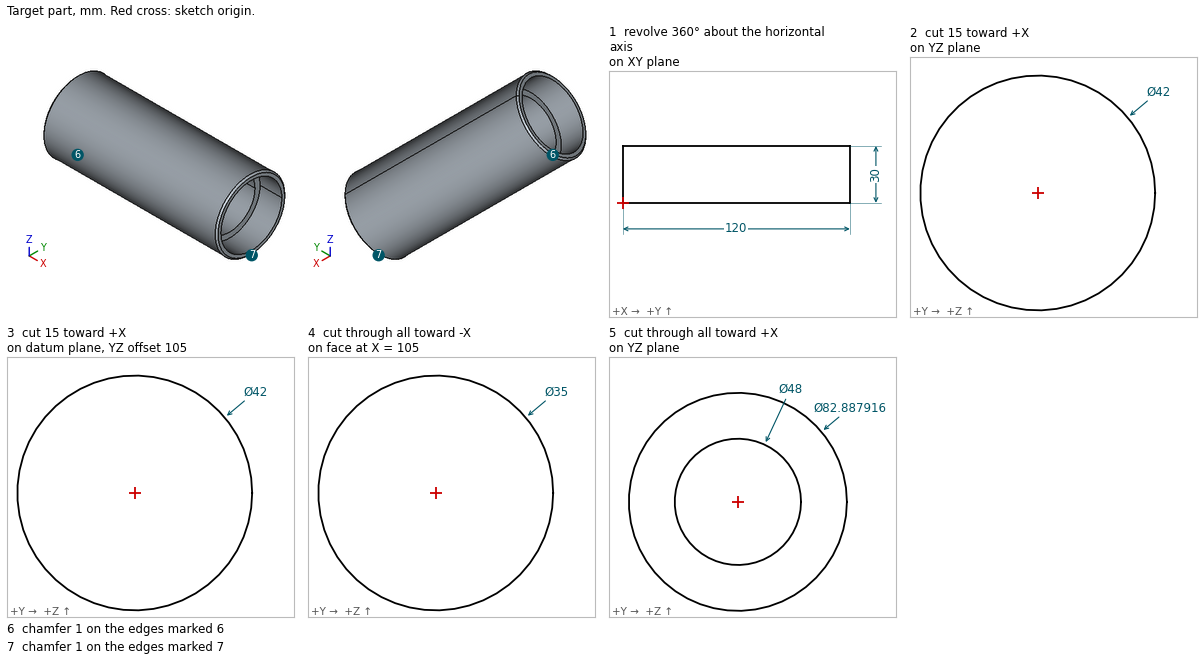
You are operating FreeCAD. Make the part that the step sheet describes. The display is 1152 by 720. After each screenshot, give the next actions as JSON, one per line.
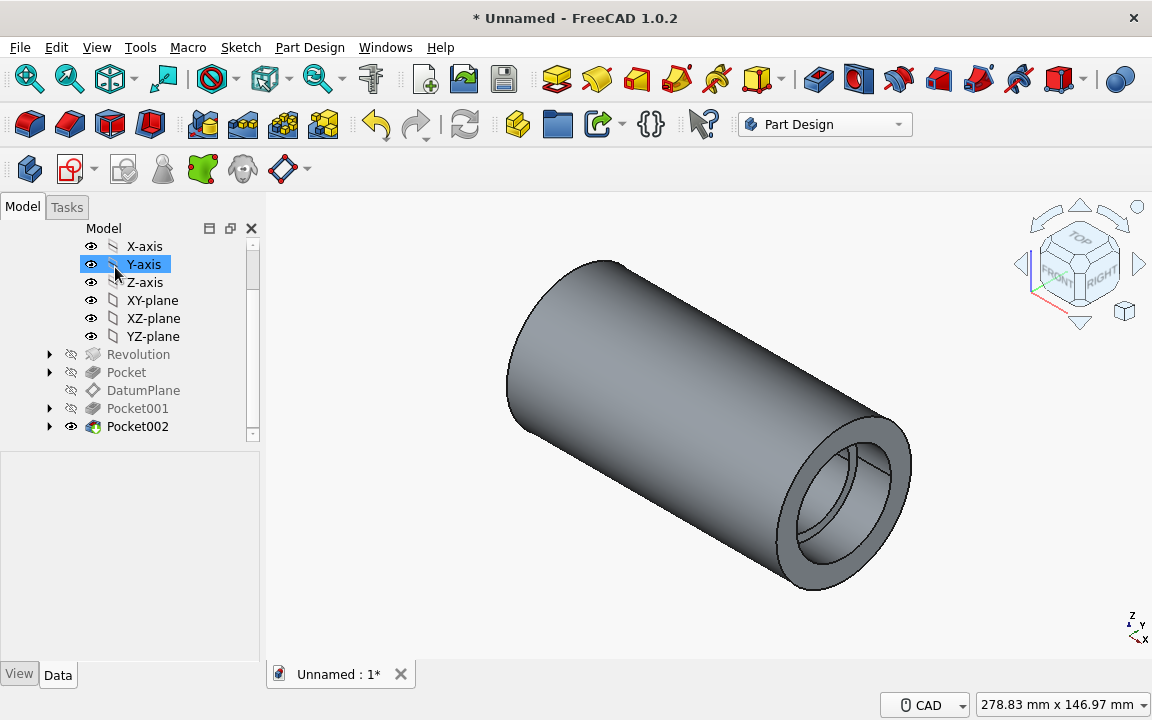
{"action": "left_click", "coordinate": [70, 170]}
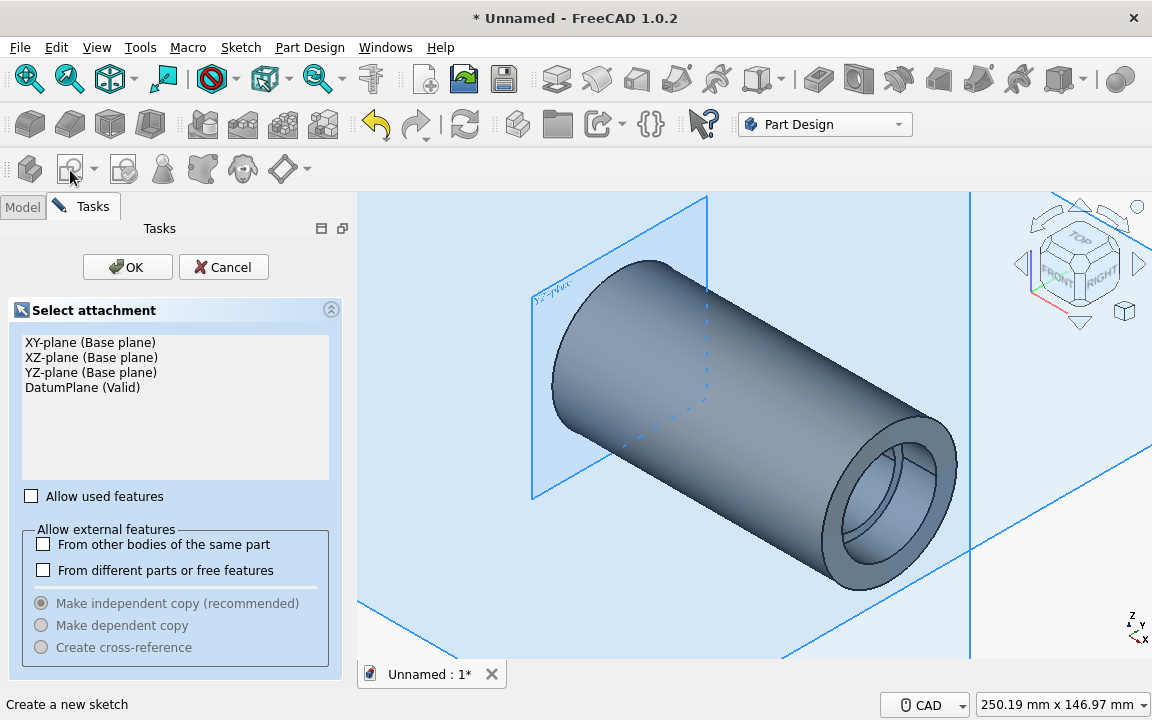
{"action": "left_click", "coordinate": [82, 372]}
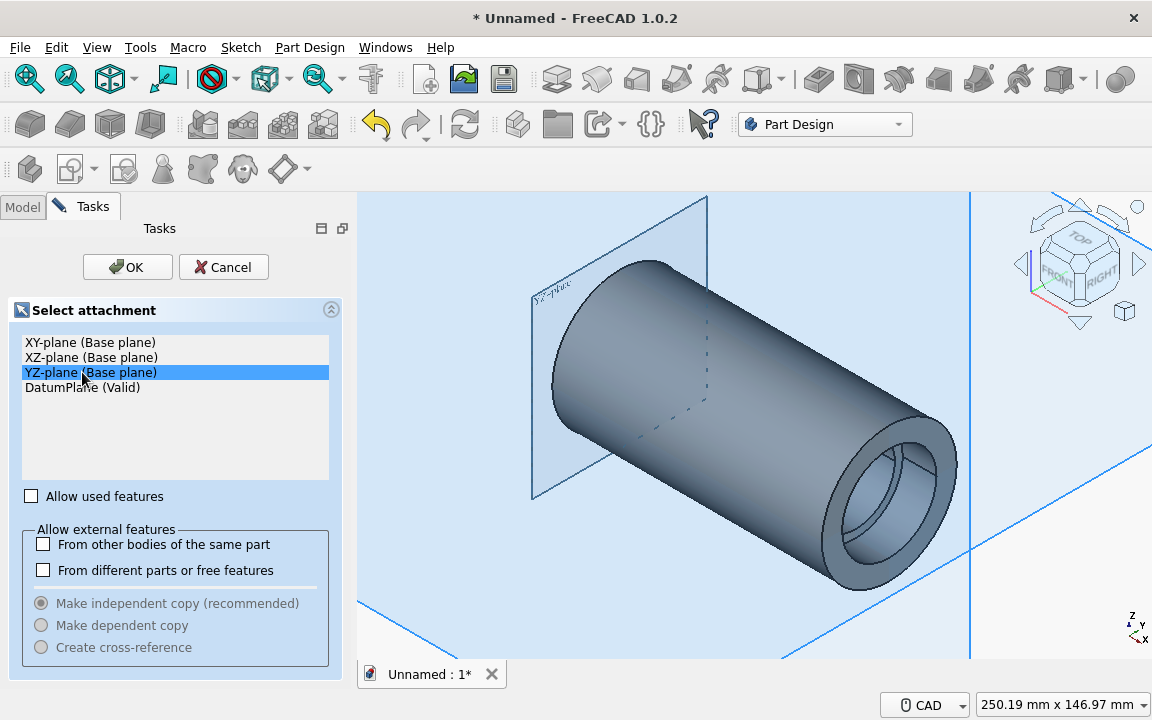
{"action": "left_click", "coordinate": [128, 267]}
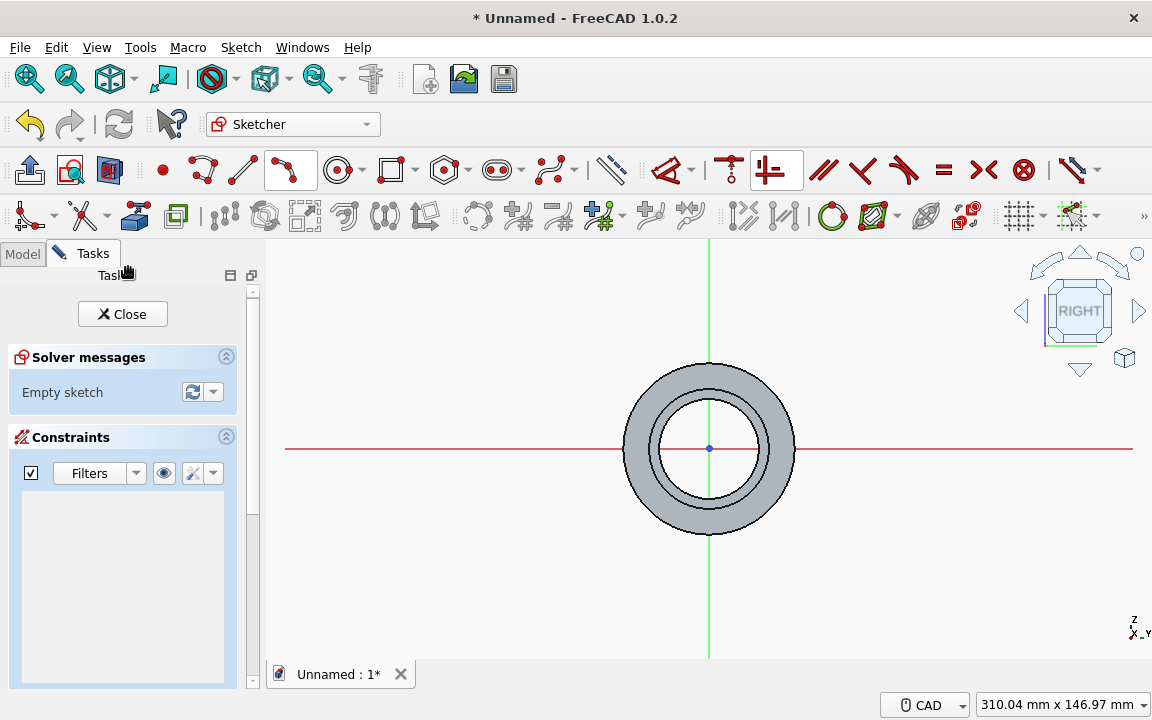
{"action": "key", "text": "q s"}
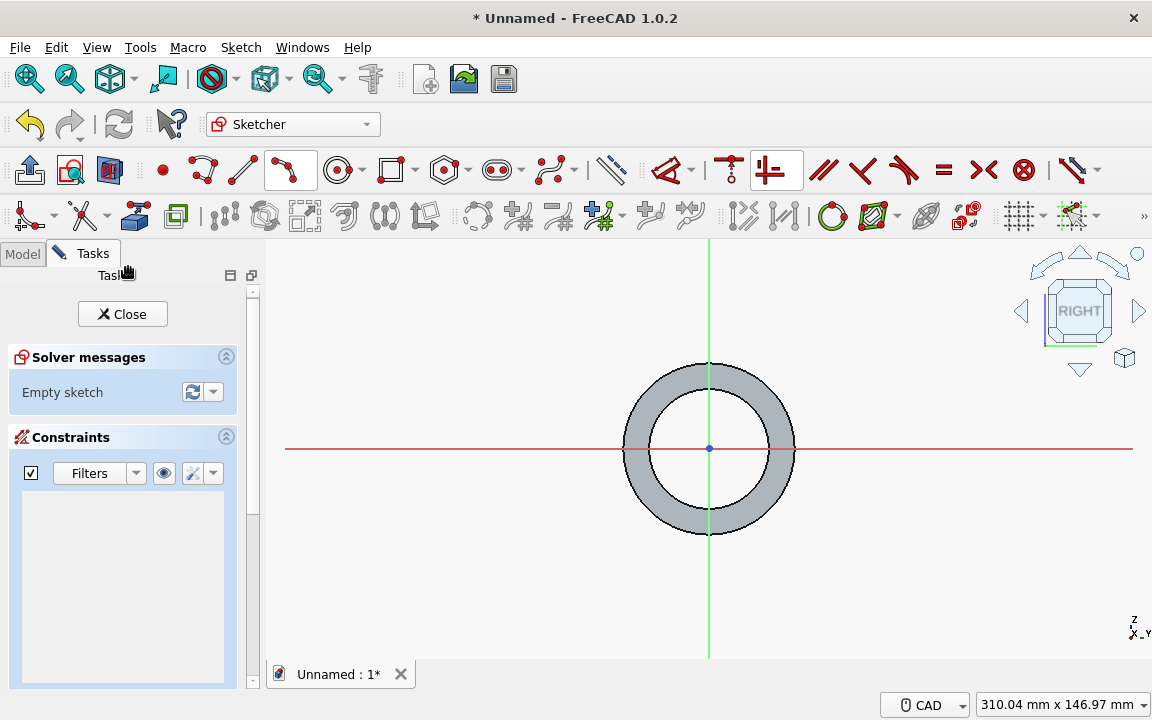
{"action": "key", "text": "g c"}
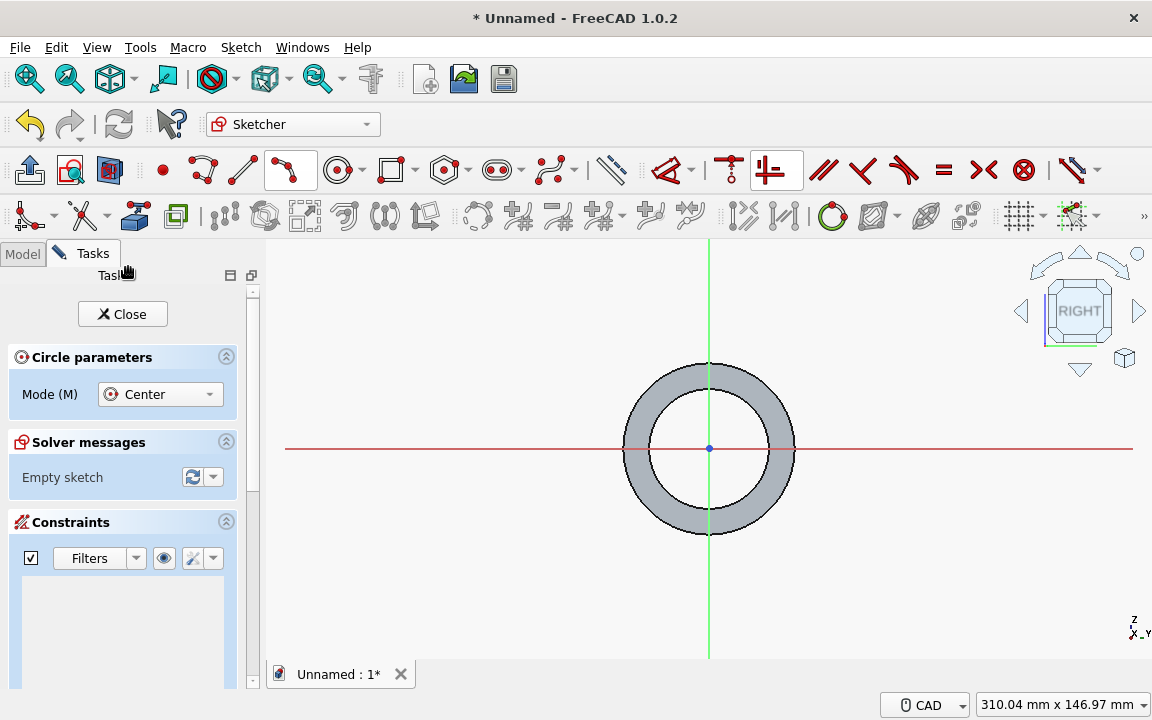
{"action": "left_click", "coordinate": [709, 449]}
{"action": "left_click", "coordinate": [793, 365]}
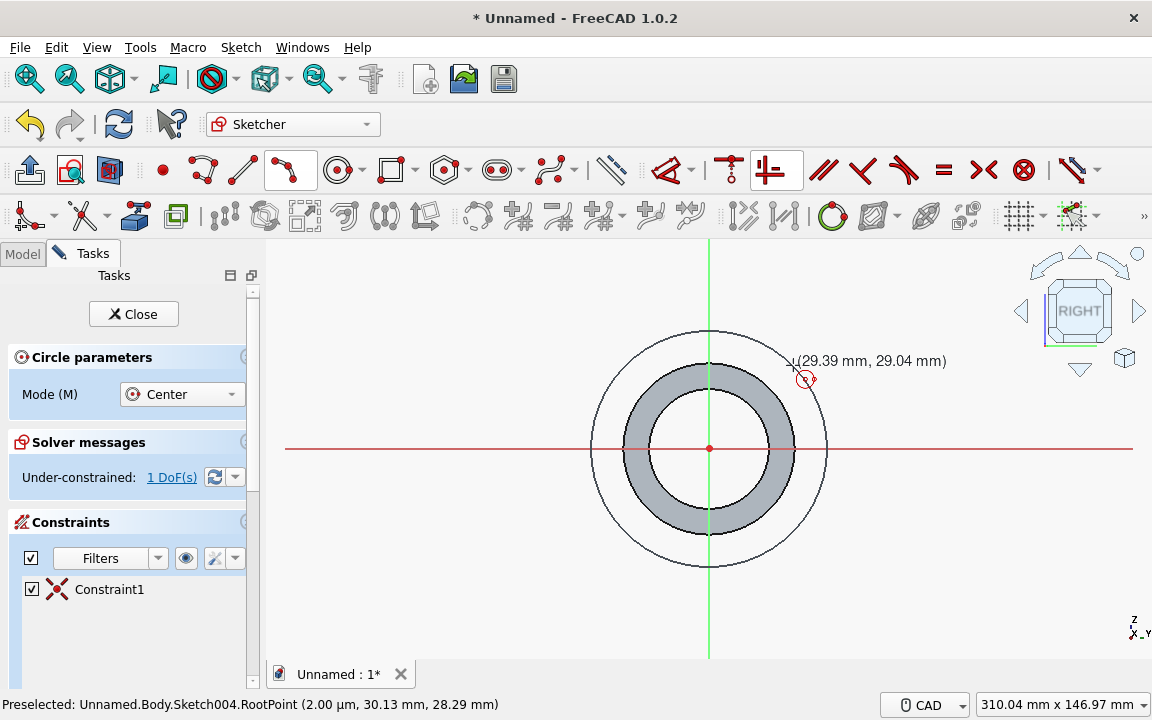
{"action": "left_click", "coordinate": [709, 449]}
{"action": "left_click", "coordinate": [757, 401]}
{"action": "key", "text": "Escape"}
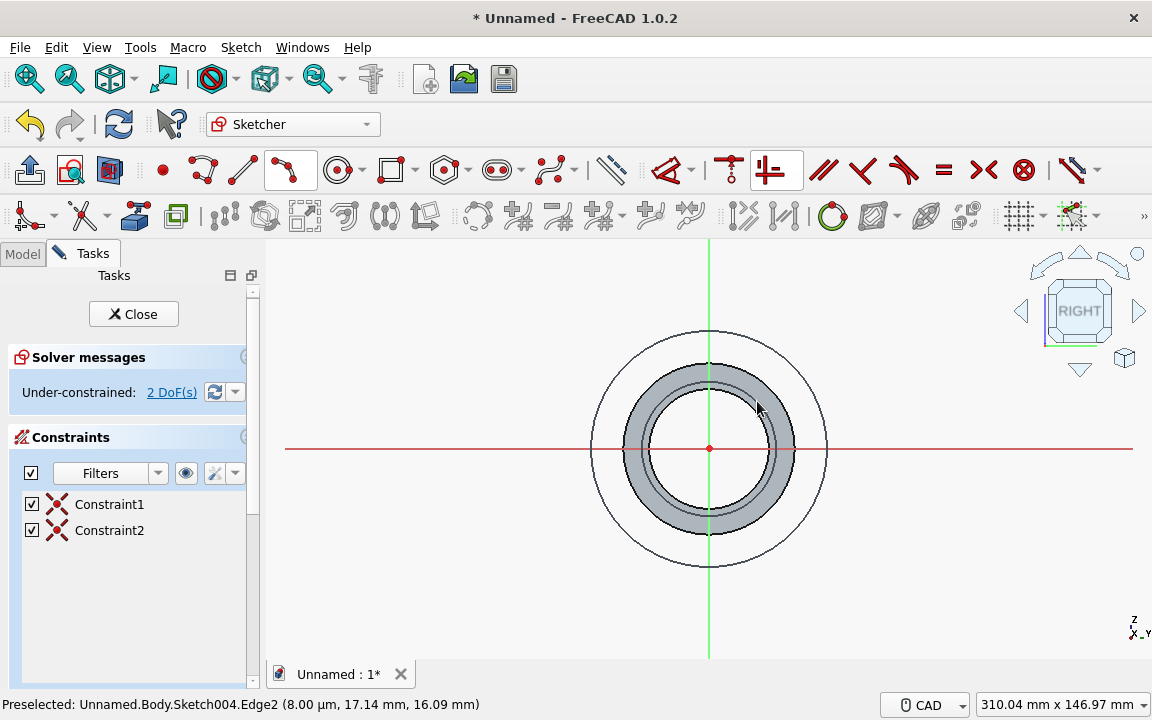
{"action": "left_click", "coordinate": [666, 170]}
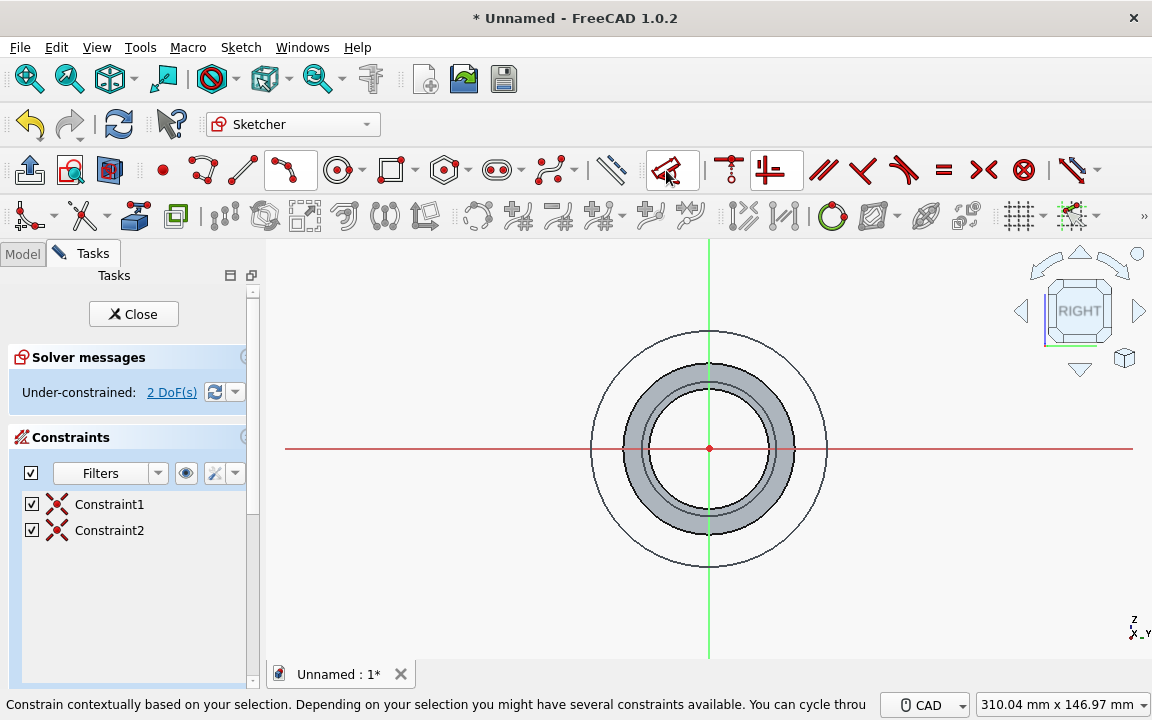
{"action": "left_click", "coordinate": [792, 365]}
{"action": "left_click", "coordinate": [814, 342]}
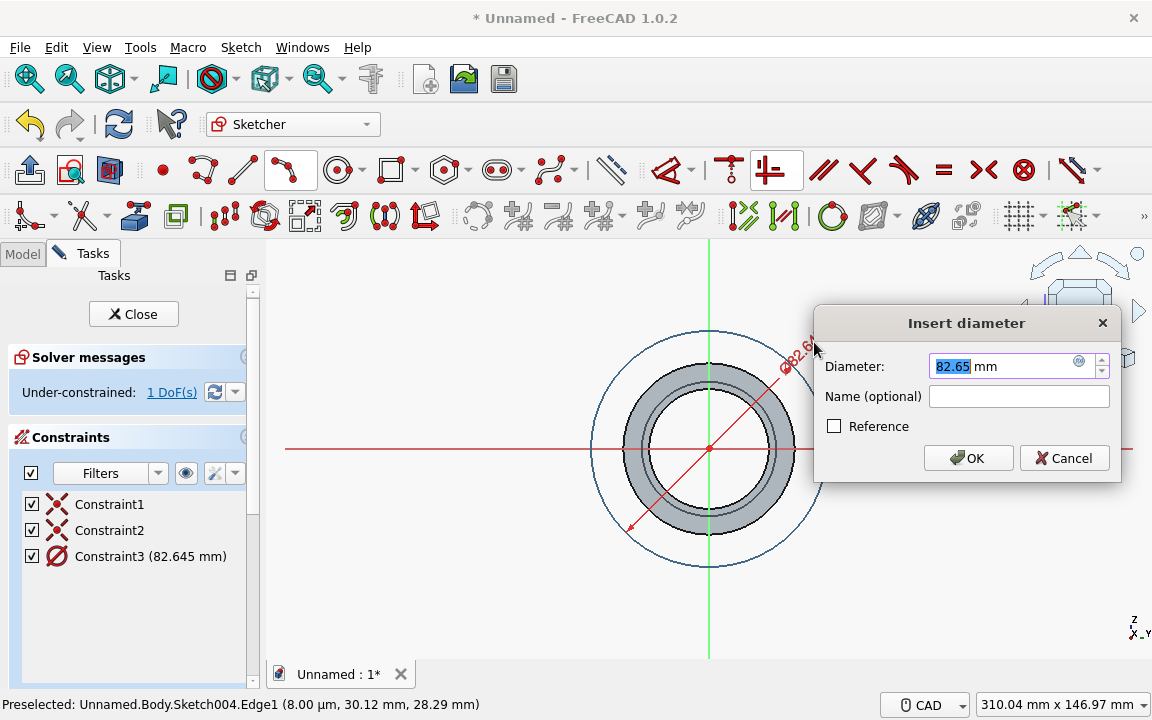
{"action": "type", "text": "82.887916"}
{"action": "key", "text": "Return"}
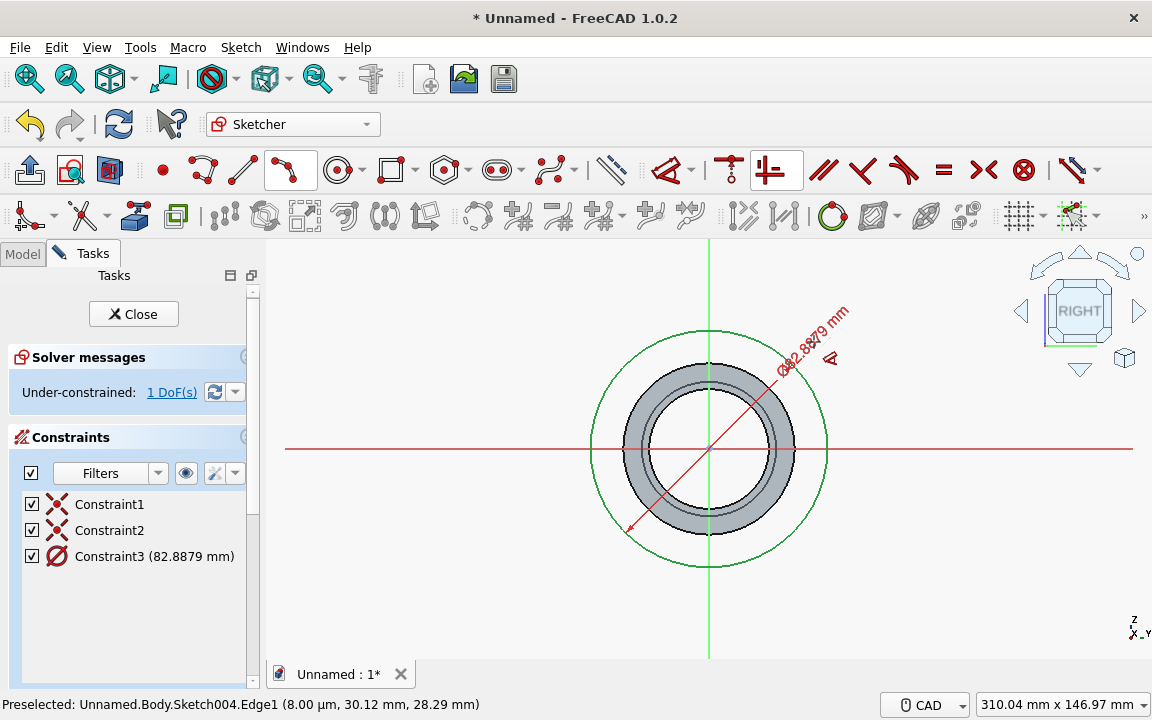
{"action": "left_click", "coordinate": [756, 401]}
{"action": "left_click", "coordinate": [778, 378]}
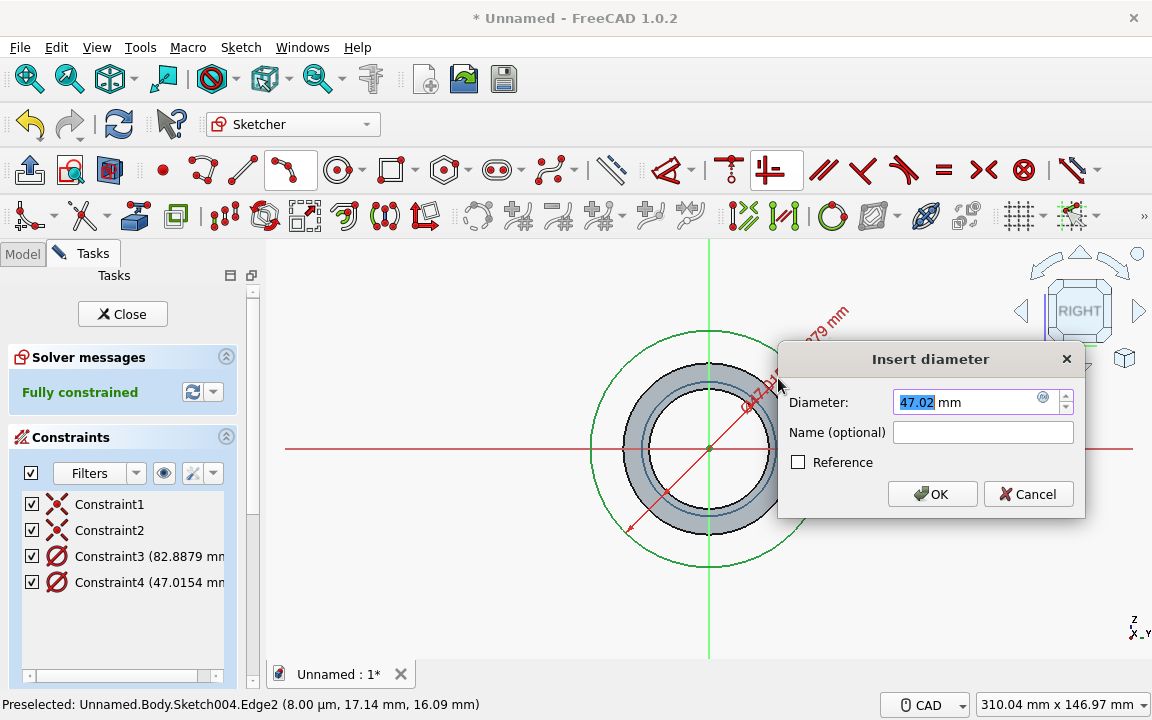
{"action": "type", "text": "48"}
{"action": "key", "text": "Return"}
{"action": "key", "text": "Escape"}